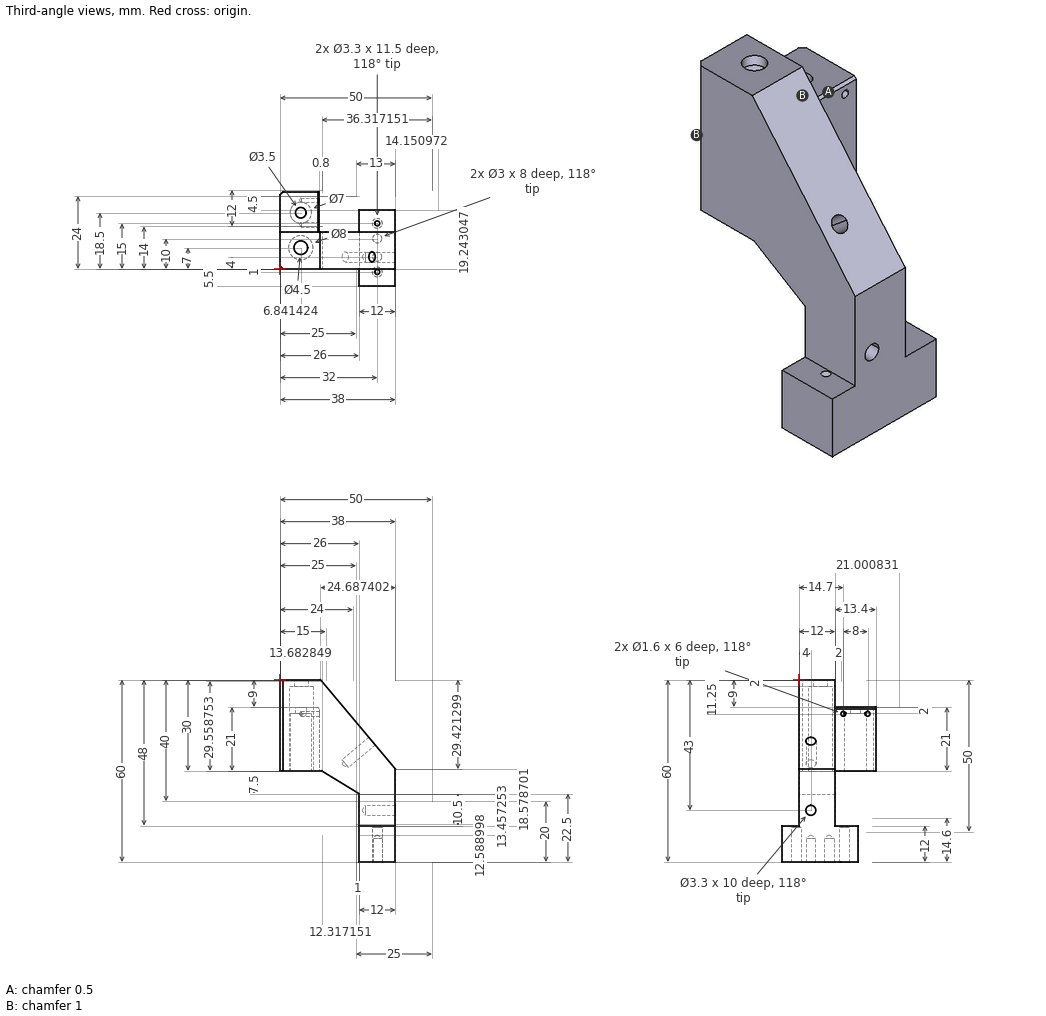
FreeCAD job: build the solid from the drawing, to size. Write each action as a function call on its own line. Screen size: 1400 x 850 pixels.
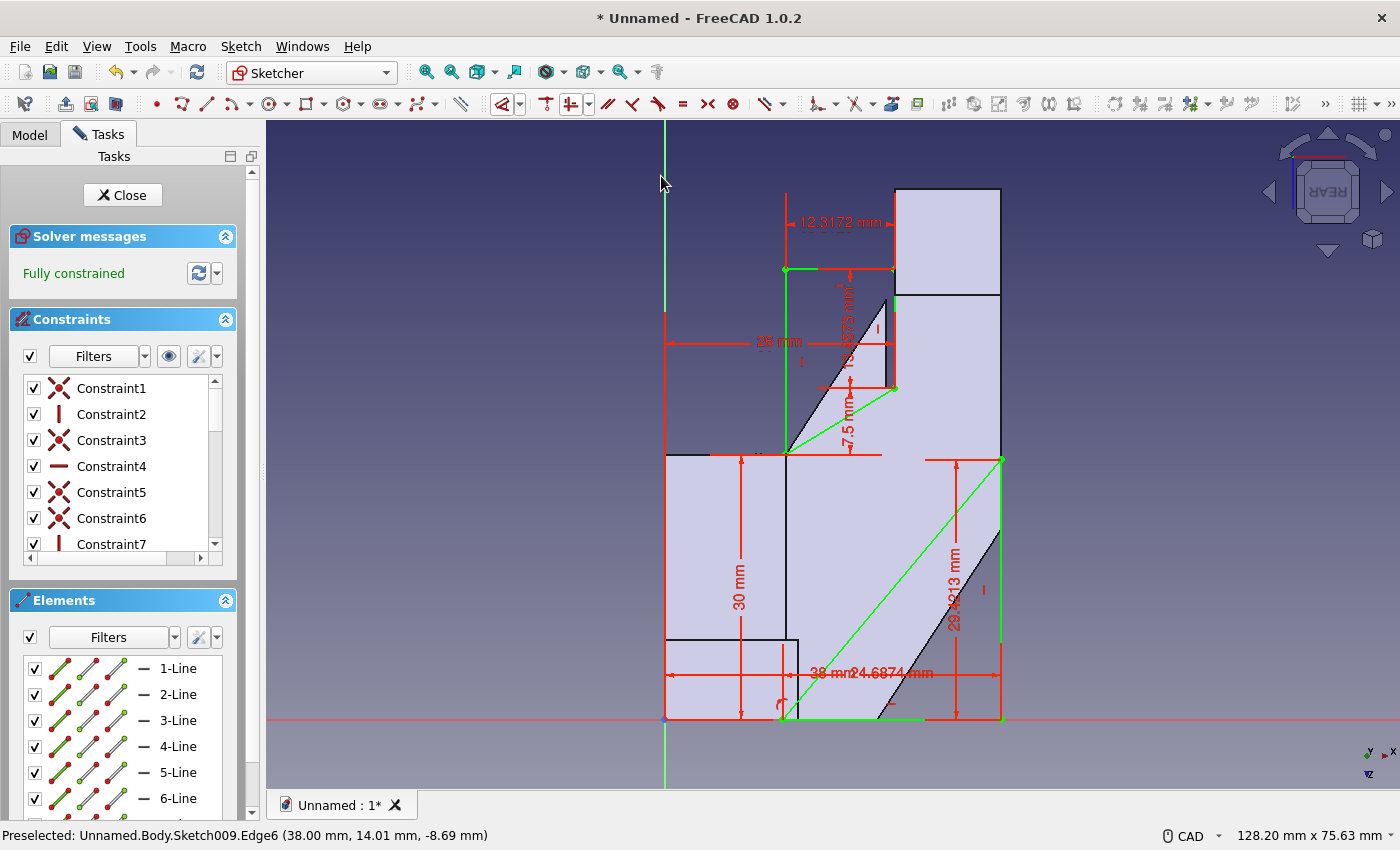
click(123, 195)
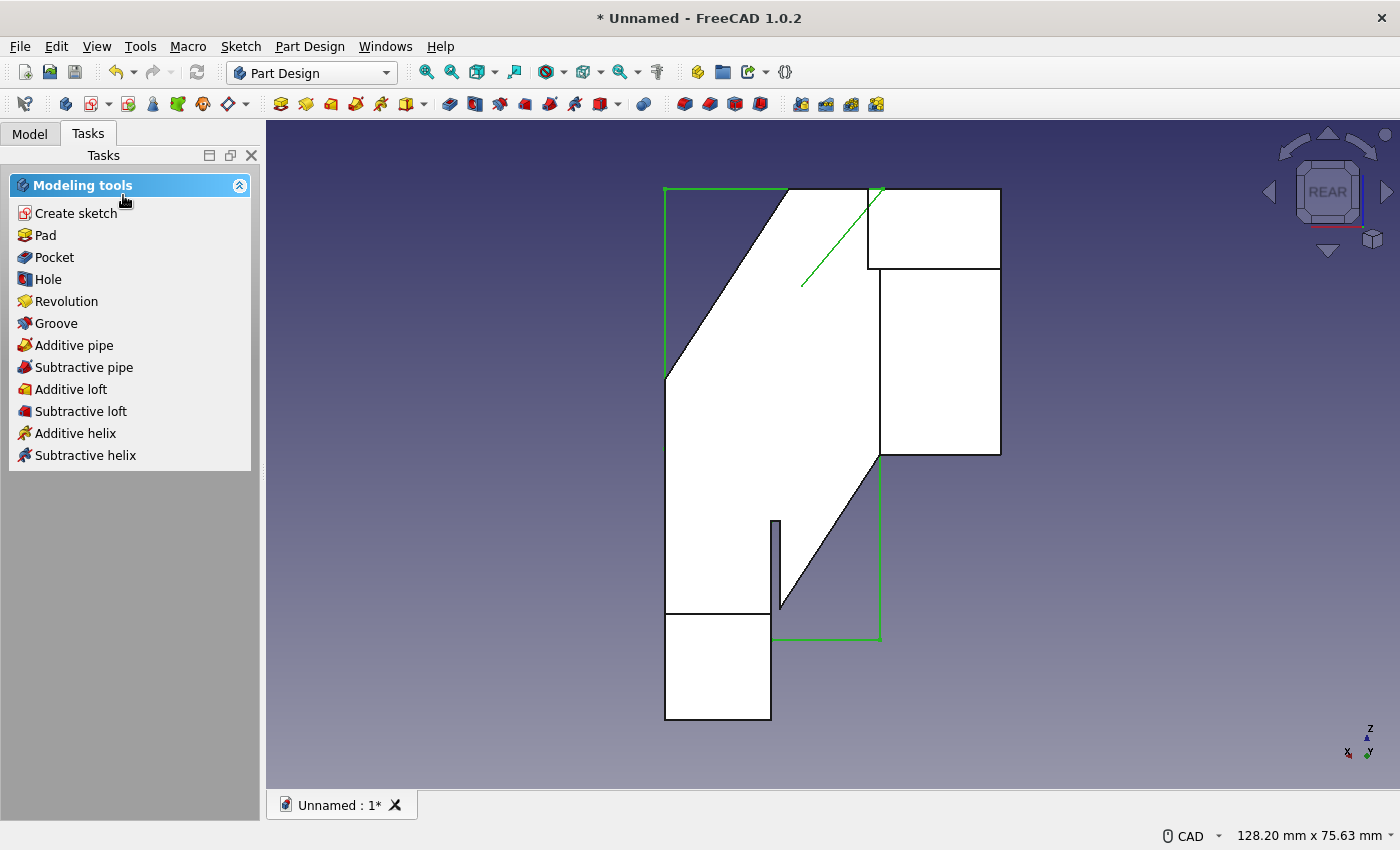
click(450, 104)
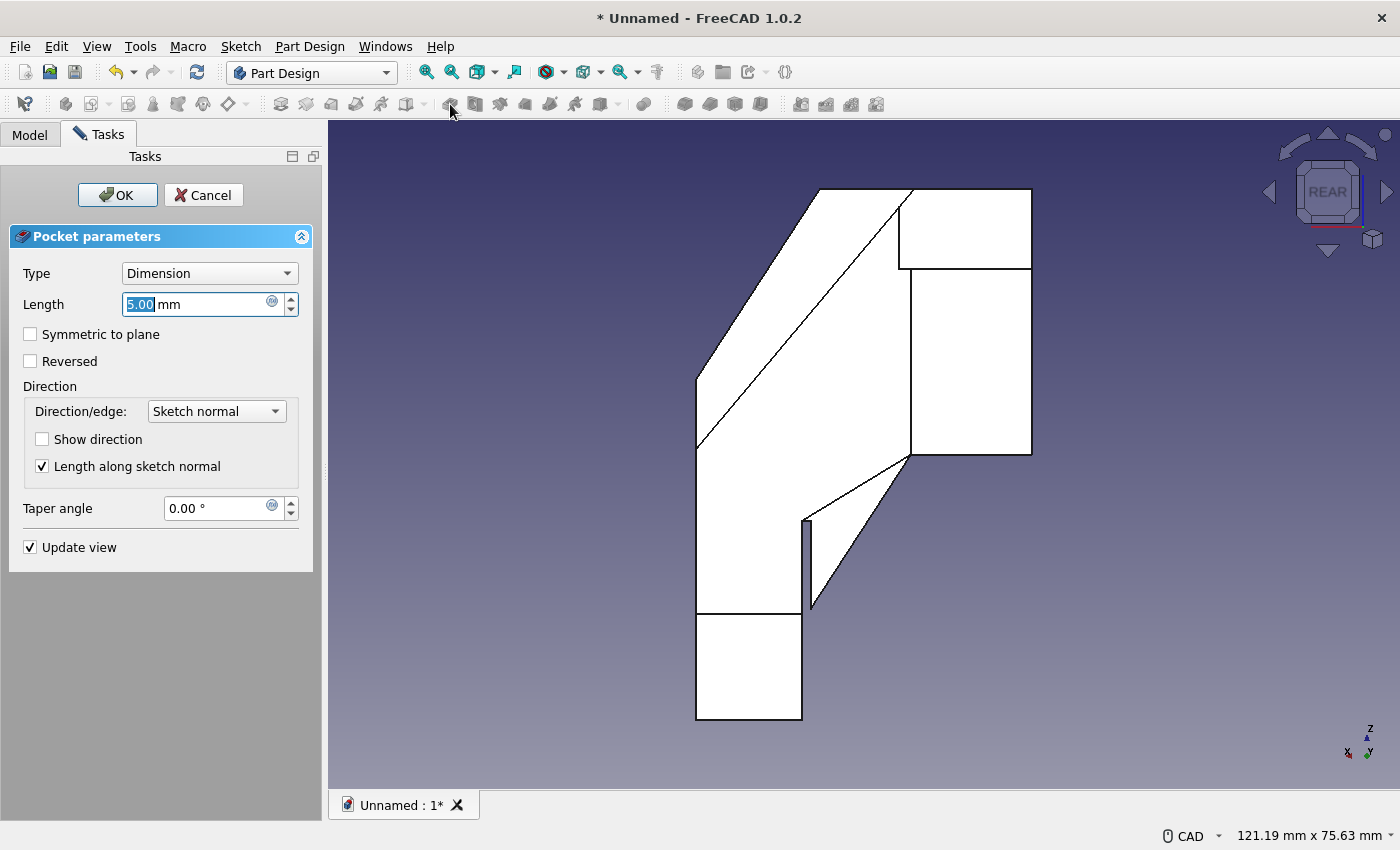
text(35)
key(Tab)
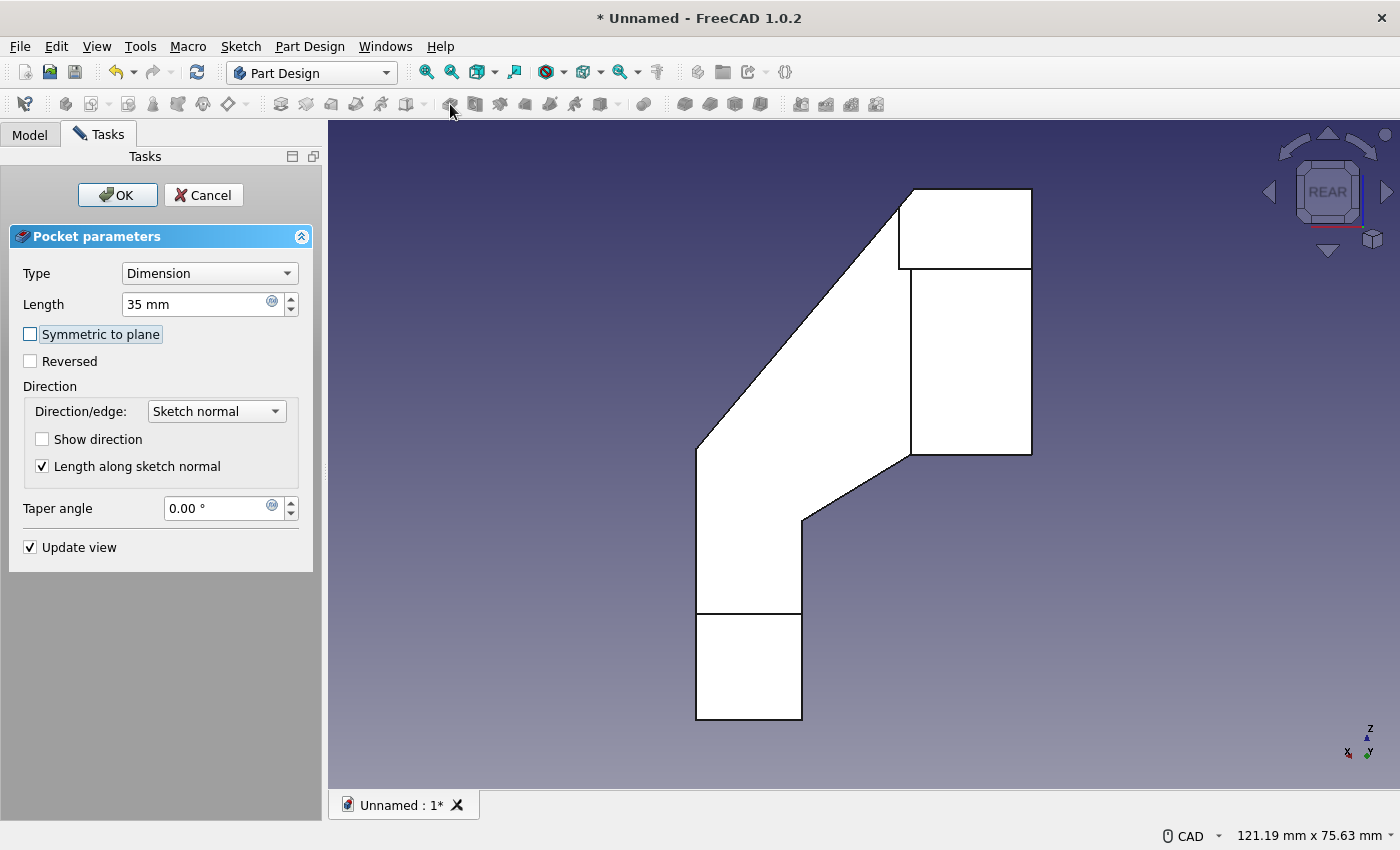
click(118, 195)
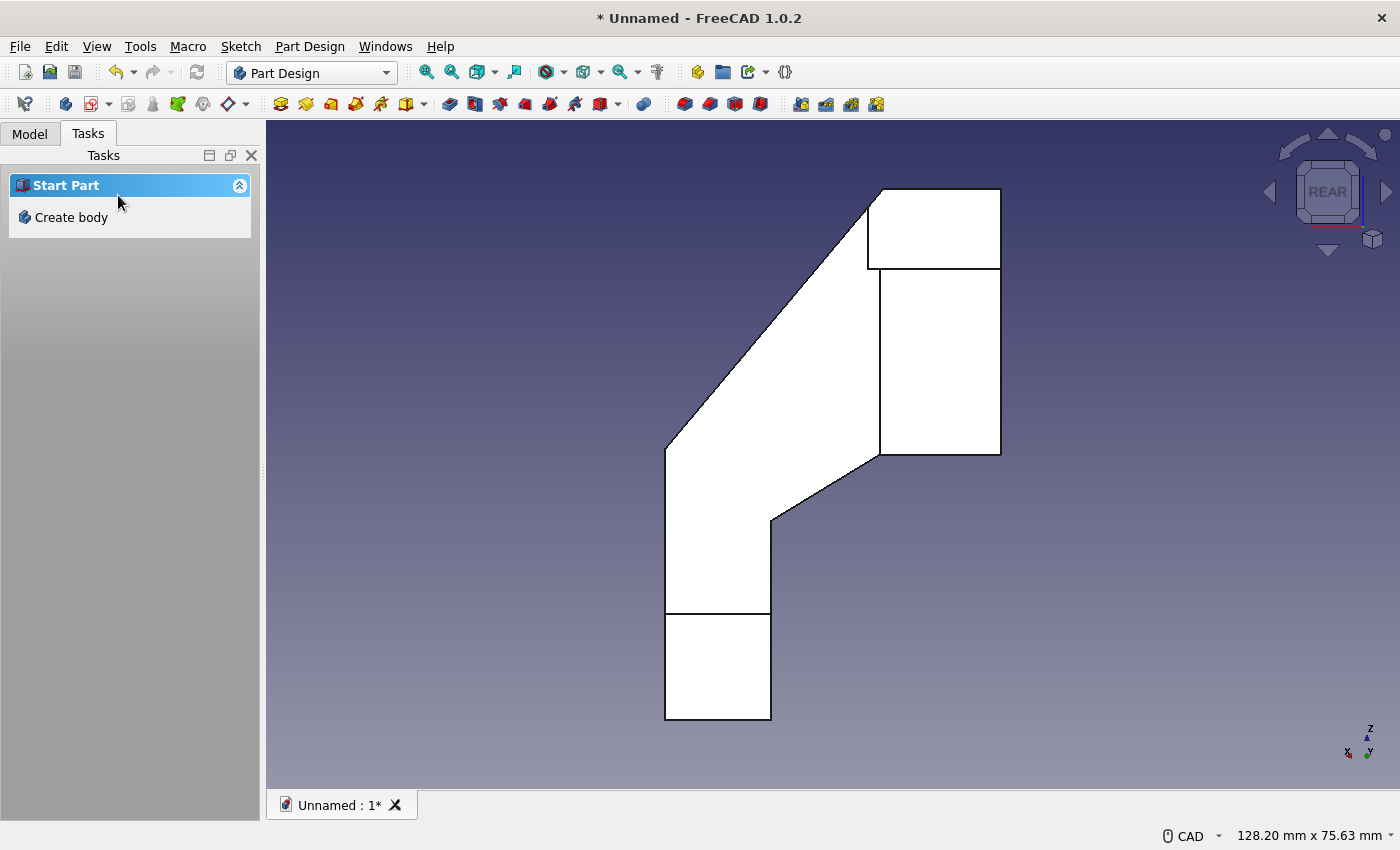
click(803, 409)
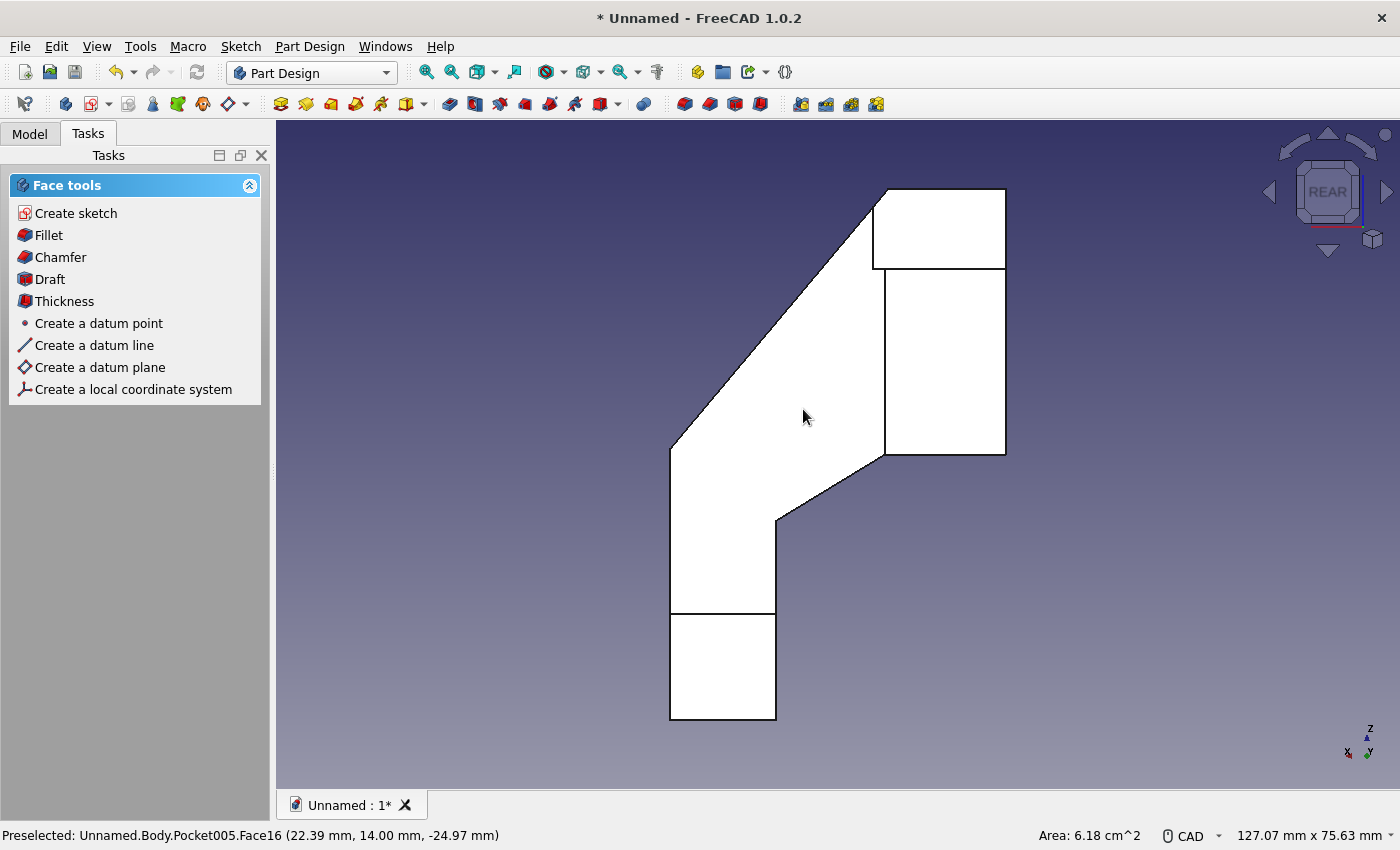
click(90, 104)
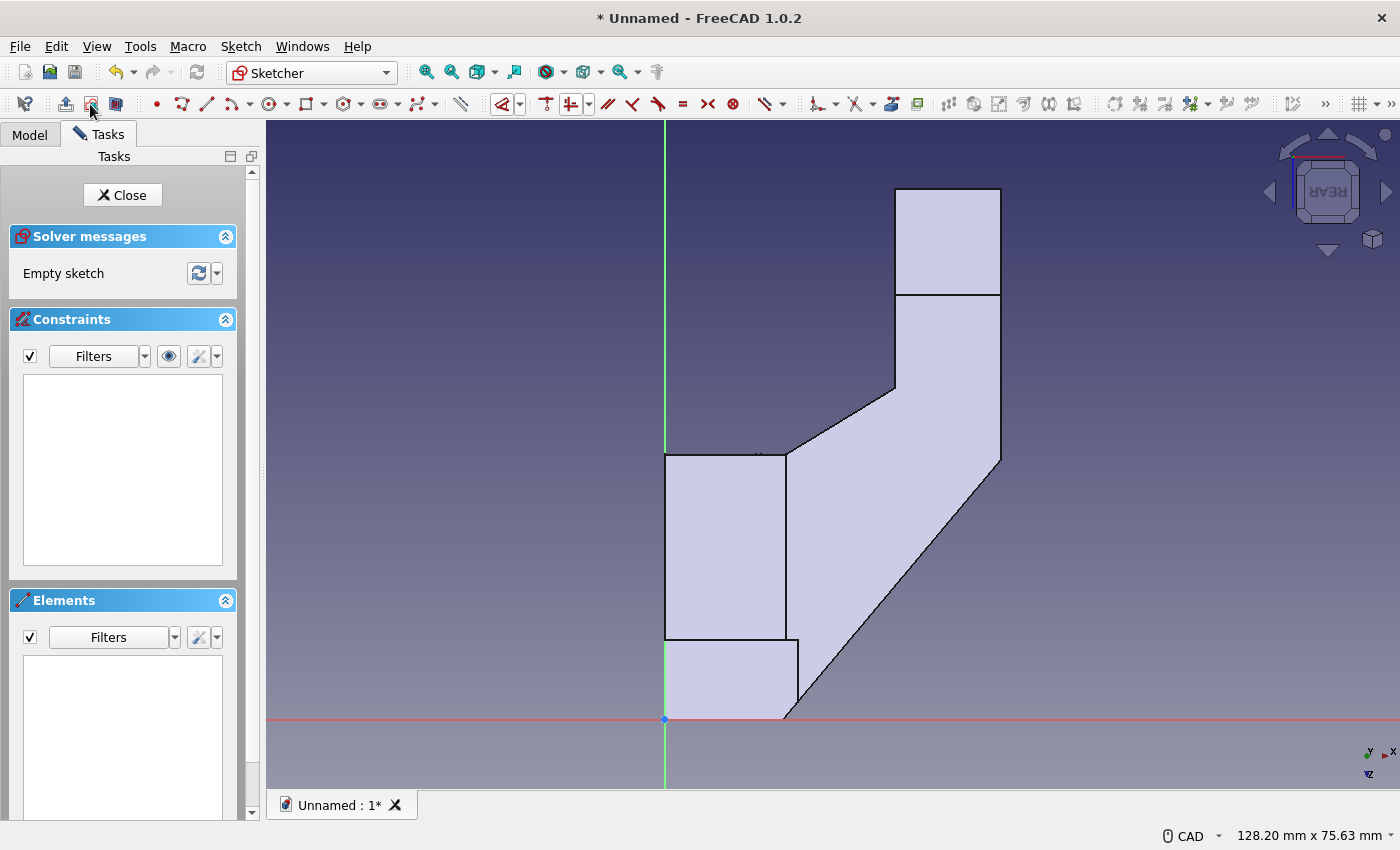
click(182, 104)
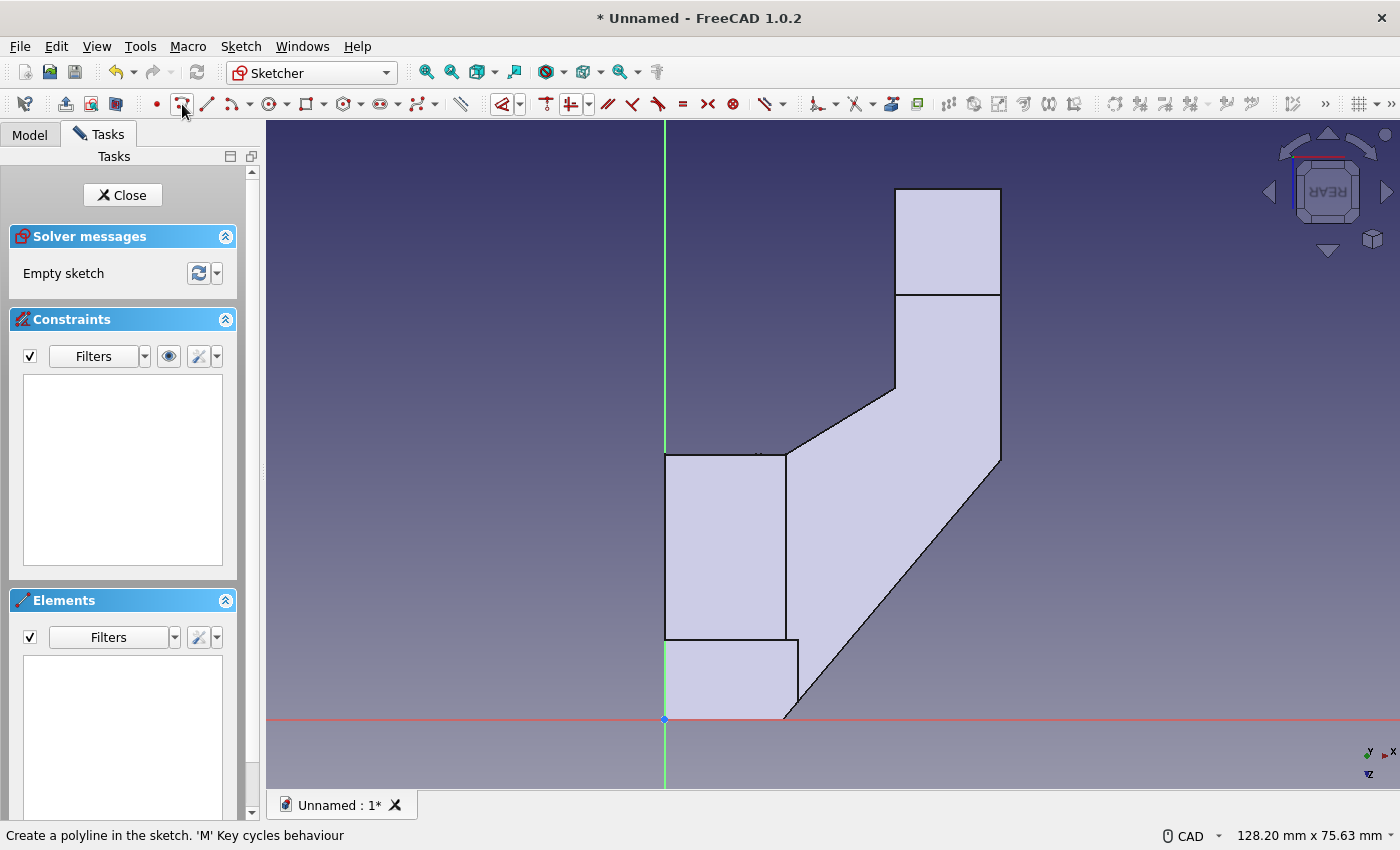
scroll(786, 716, up, 8)